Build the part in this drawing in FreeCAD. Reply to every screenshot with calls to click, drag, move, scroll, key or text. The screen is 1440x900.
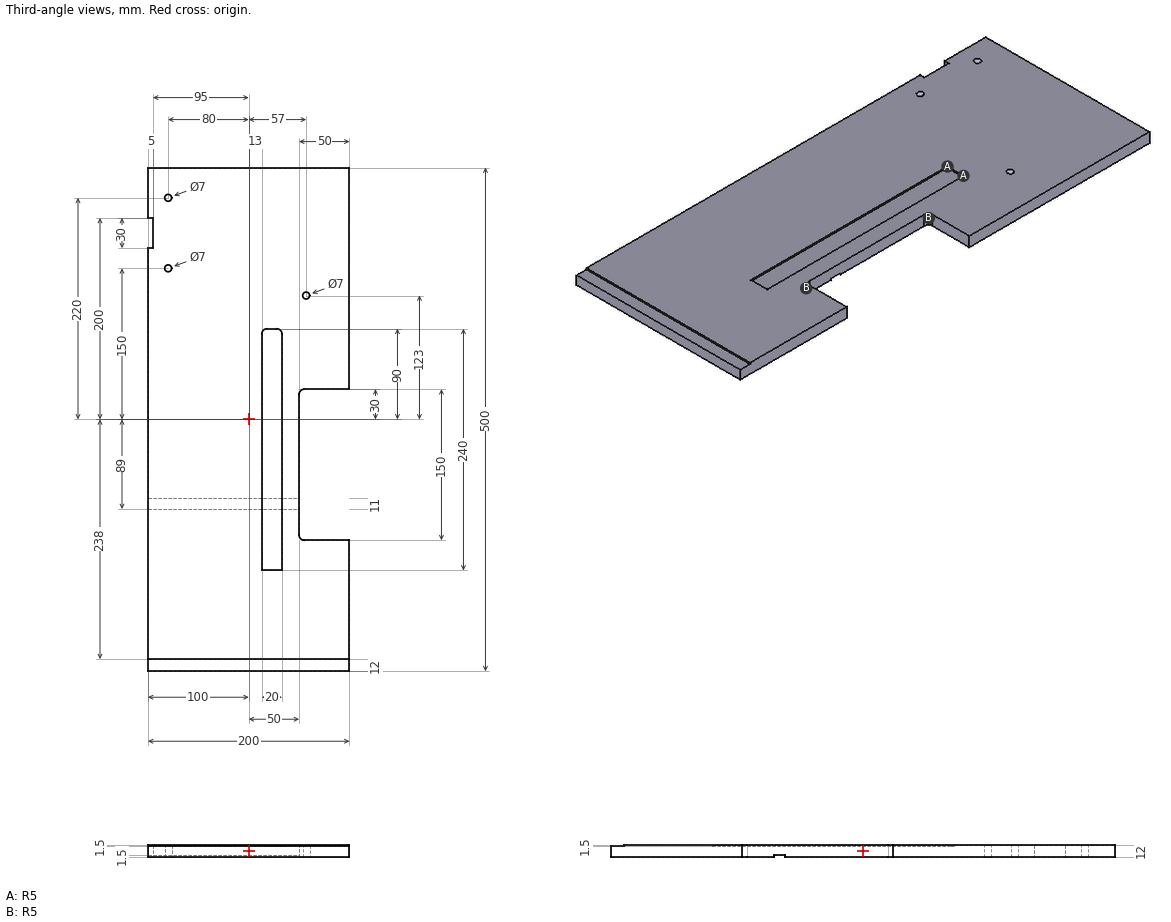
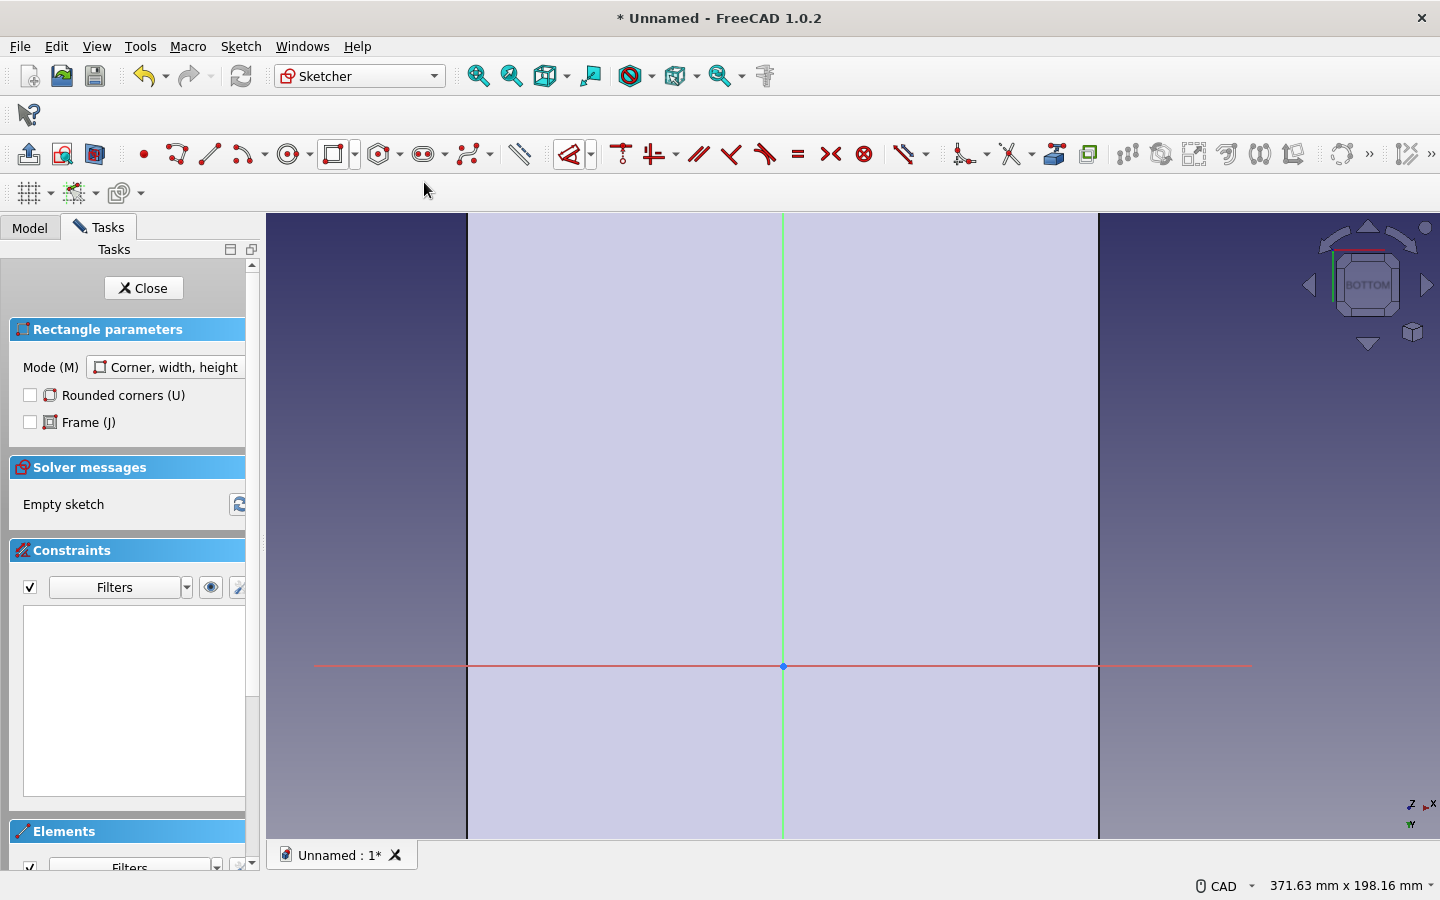
click(467, 385)
move(1099, 420)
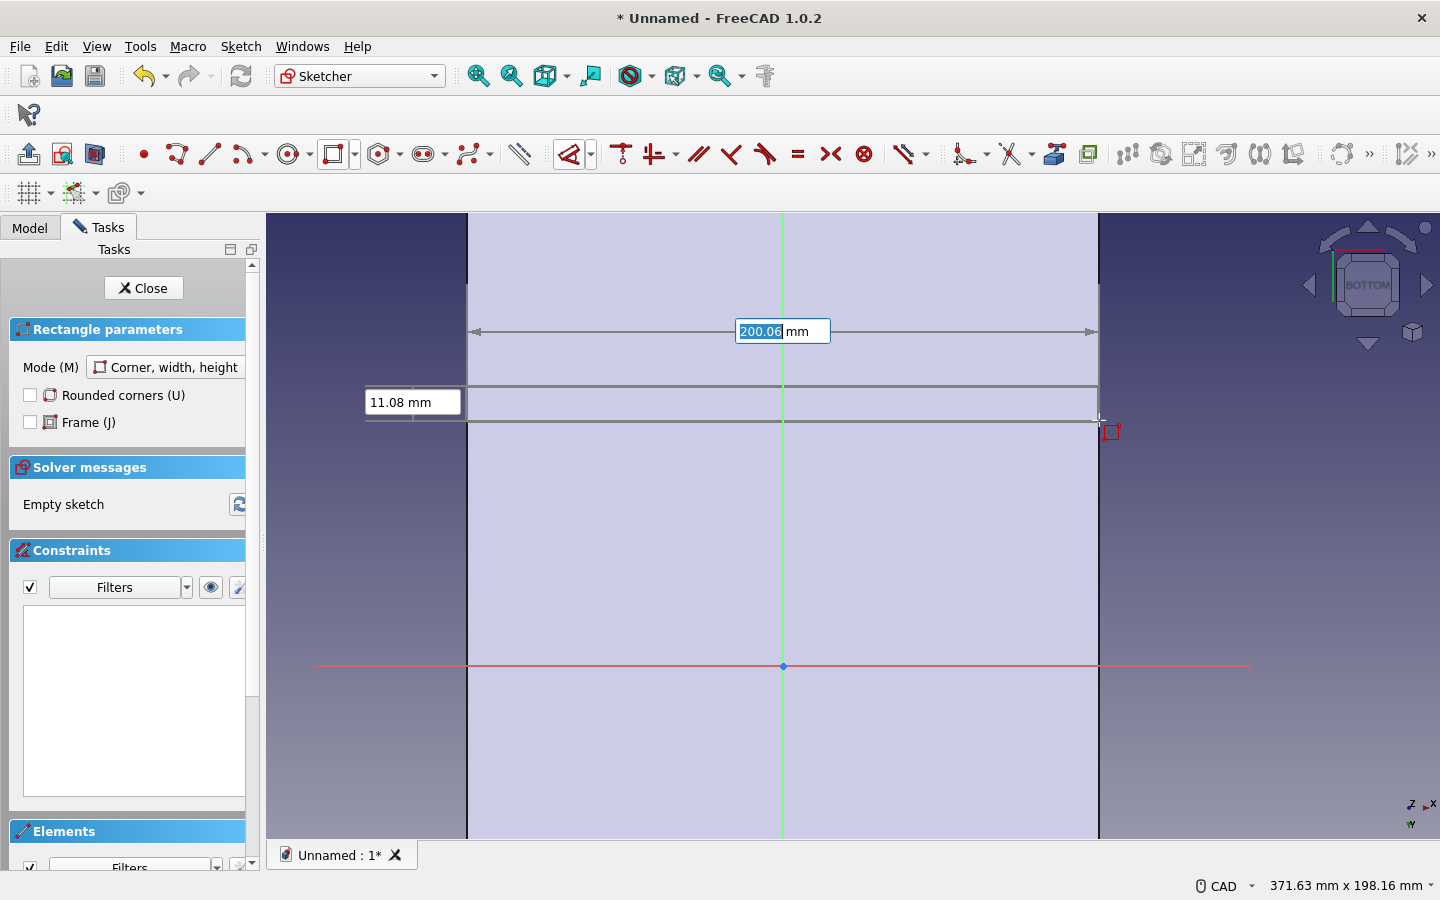
text(200)
key(Tab)
text(11)
key(Return)
key(Escape)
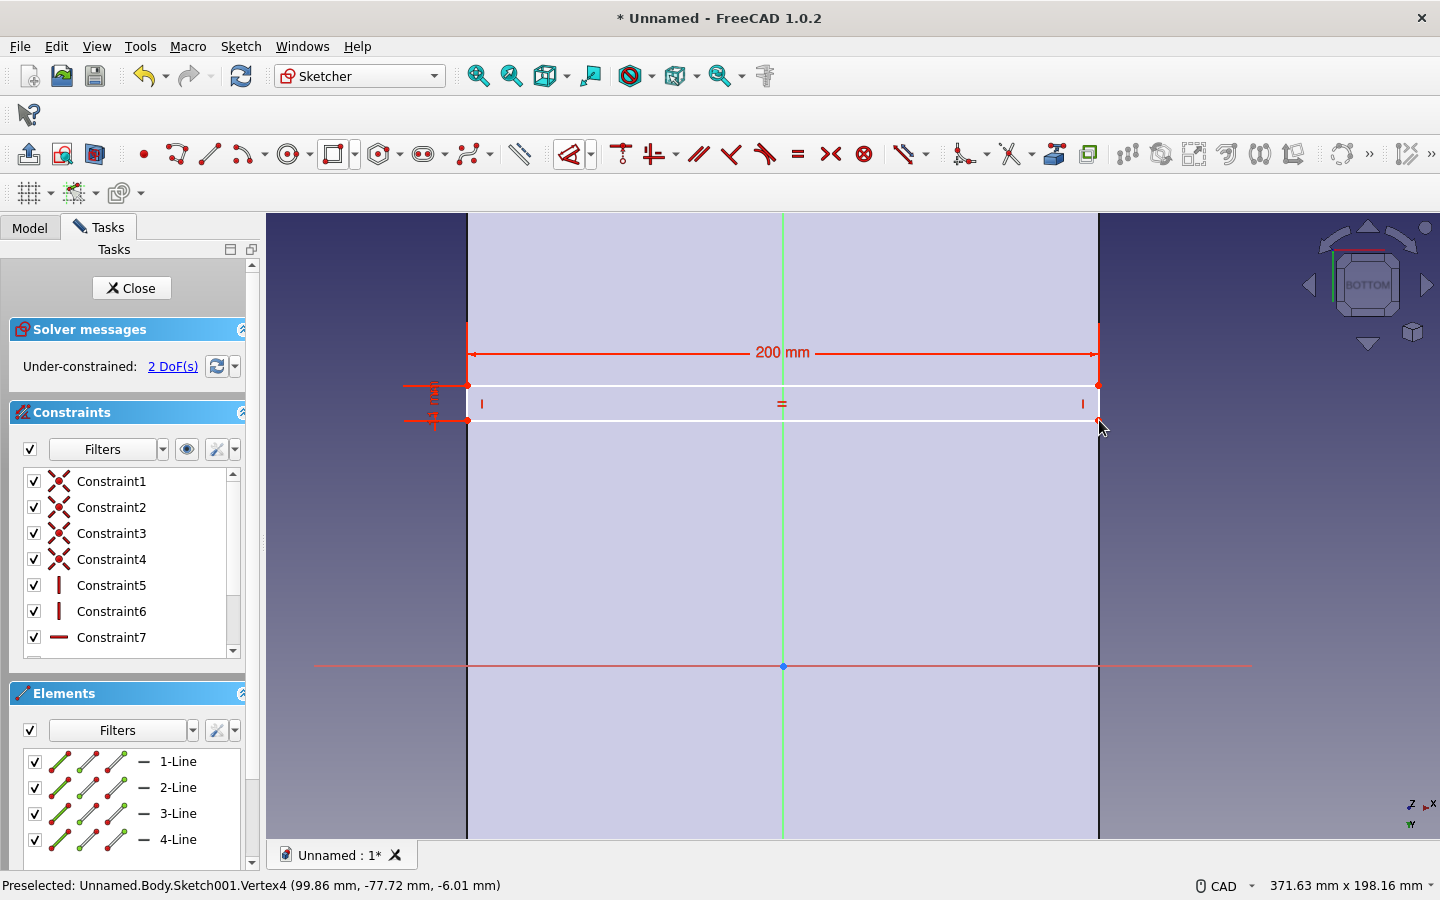
key(d)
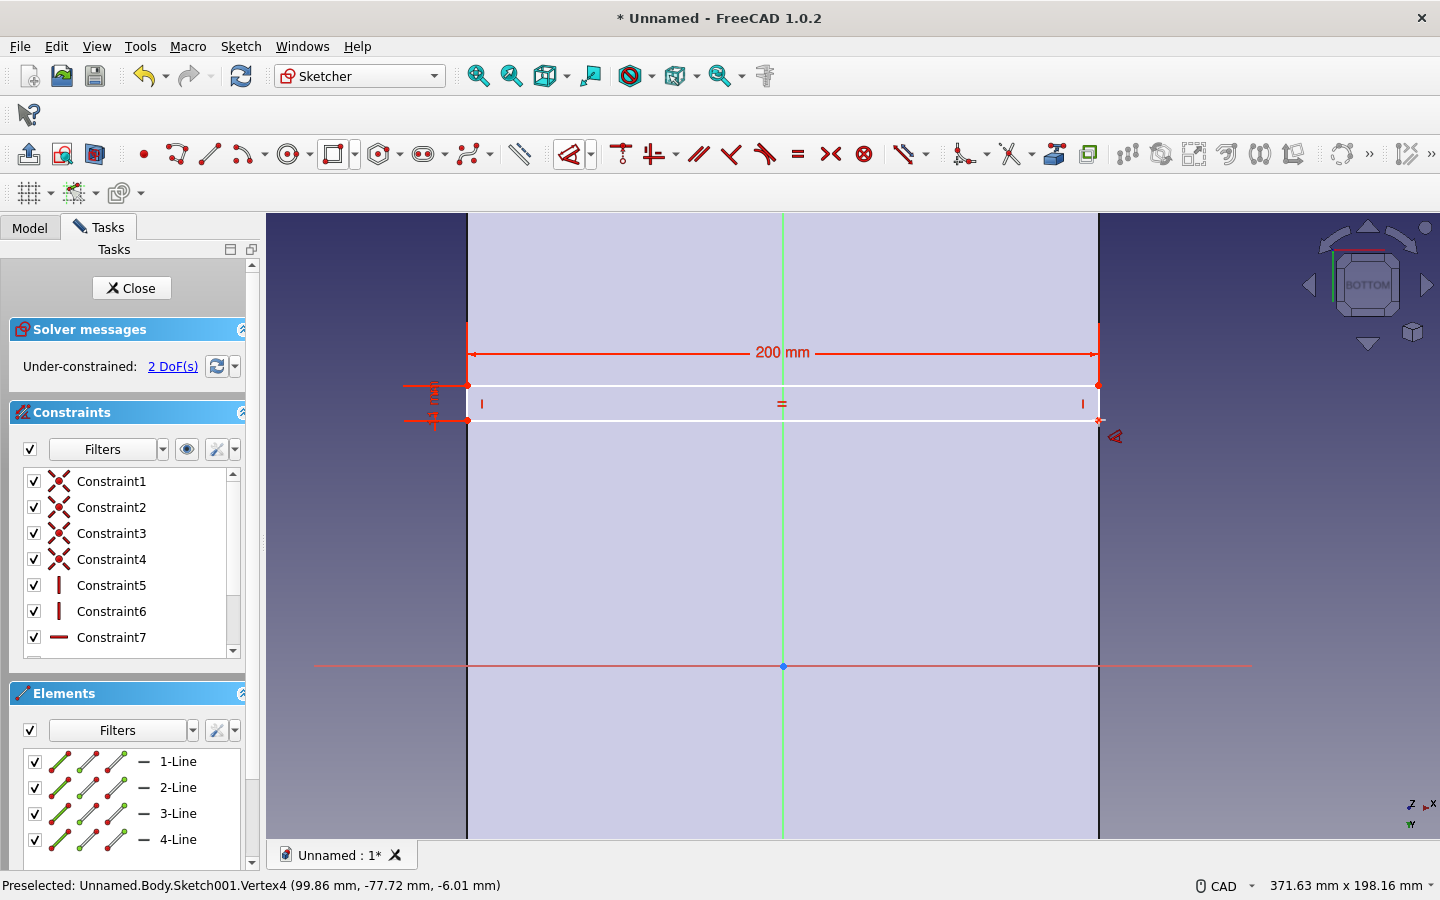
click(467, 386)
click(433, 526)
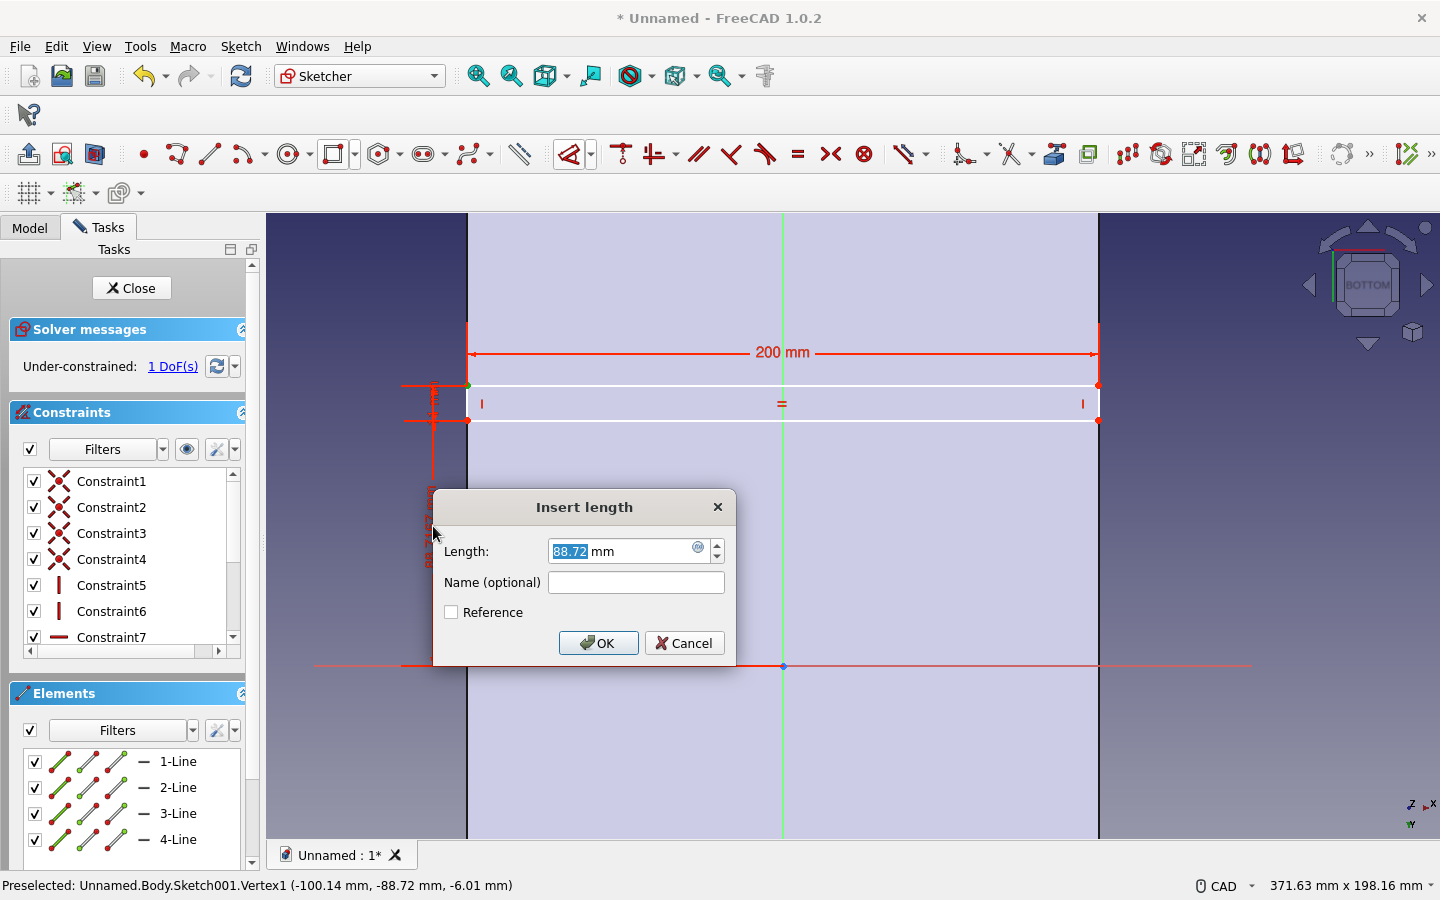
text(89)
key(Return)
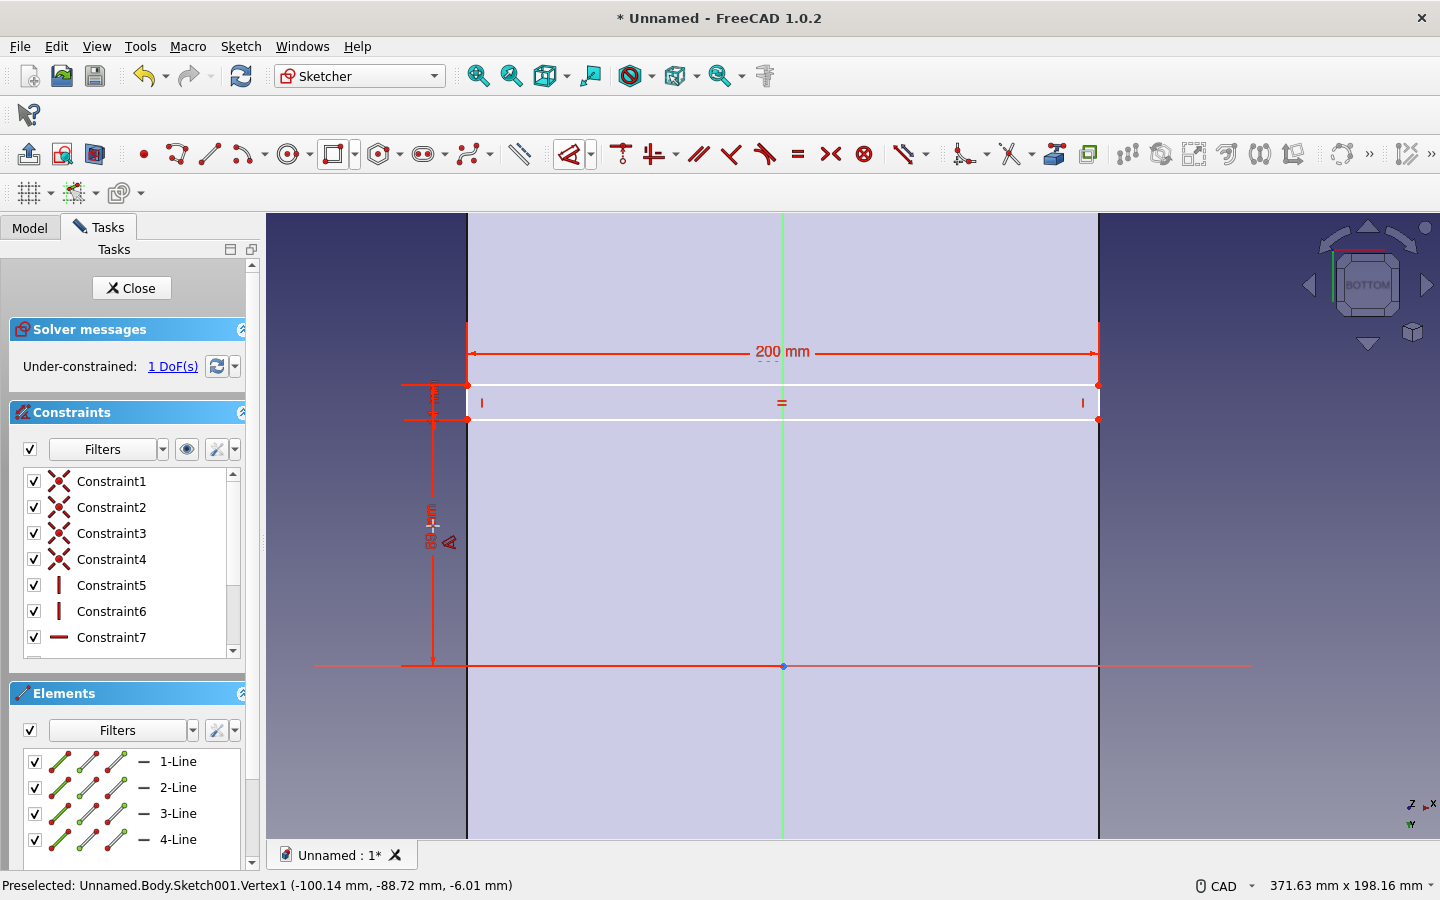
click(467, 385)
click(625, 700)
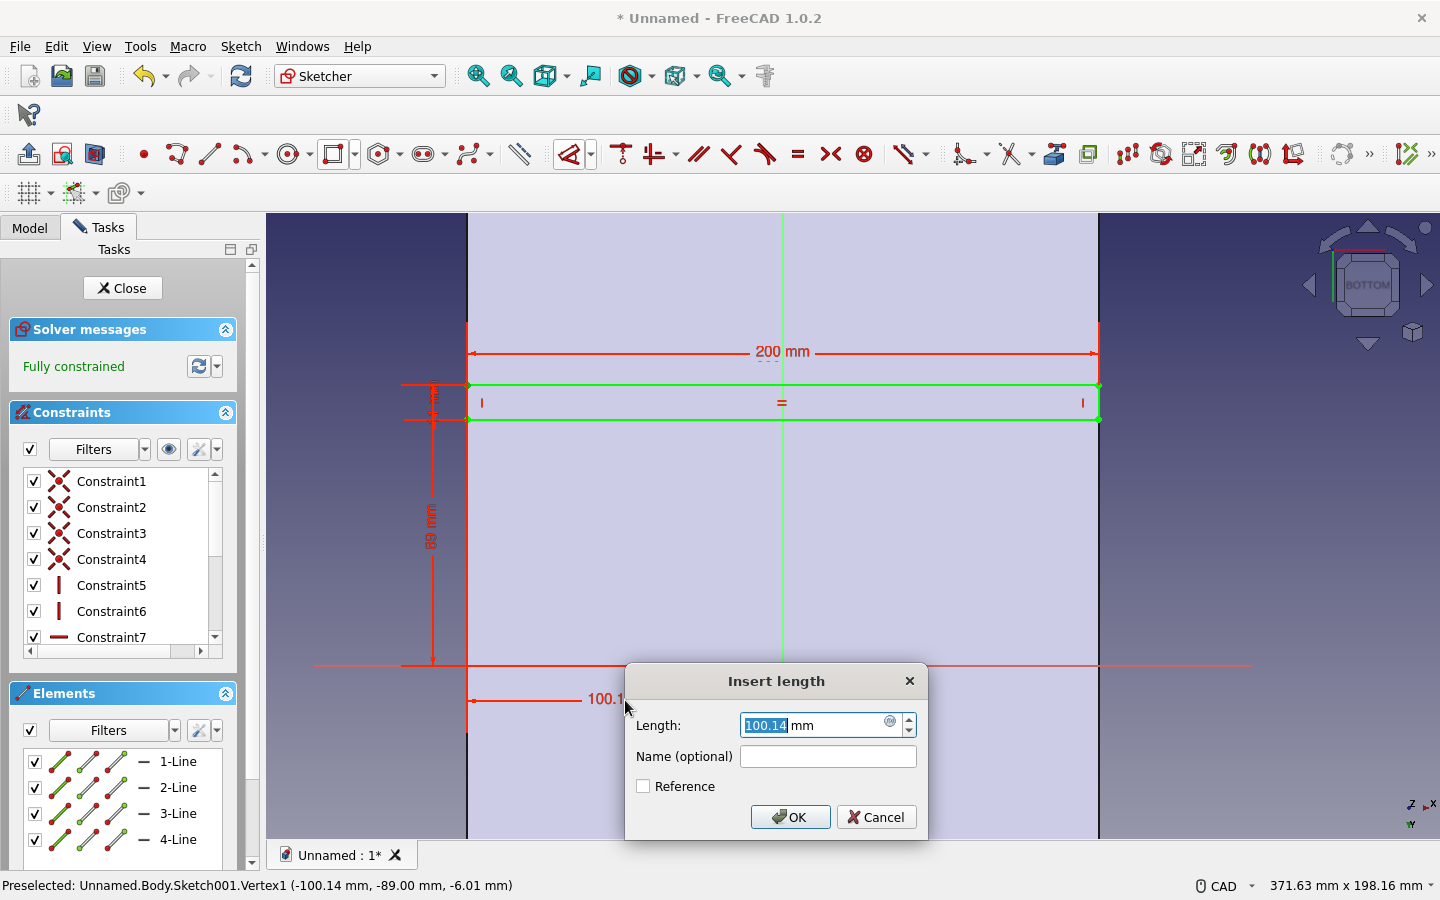
text(100)
key(Return)
key(Escape)